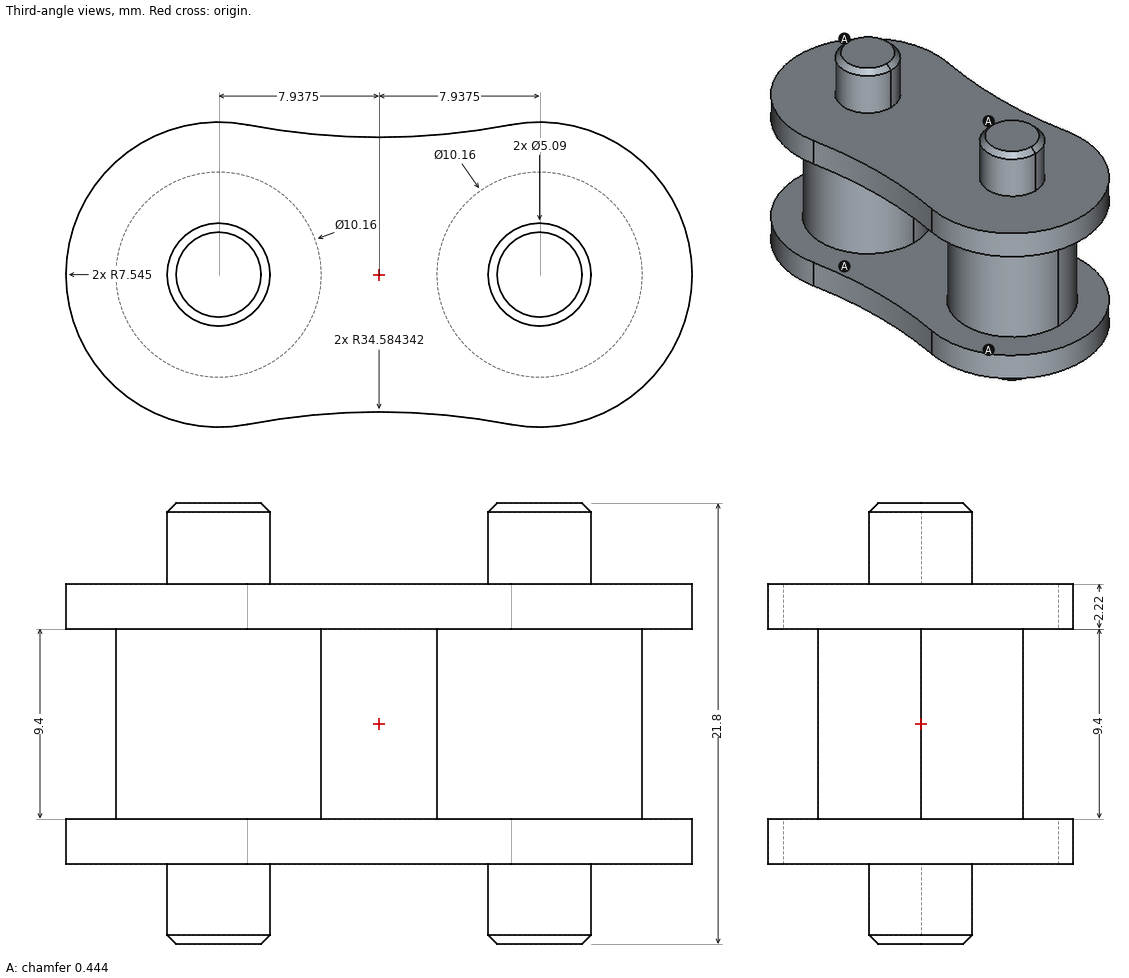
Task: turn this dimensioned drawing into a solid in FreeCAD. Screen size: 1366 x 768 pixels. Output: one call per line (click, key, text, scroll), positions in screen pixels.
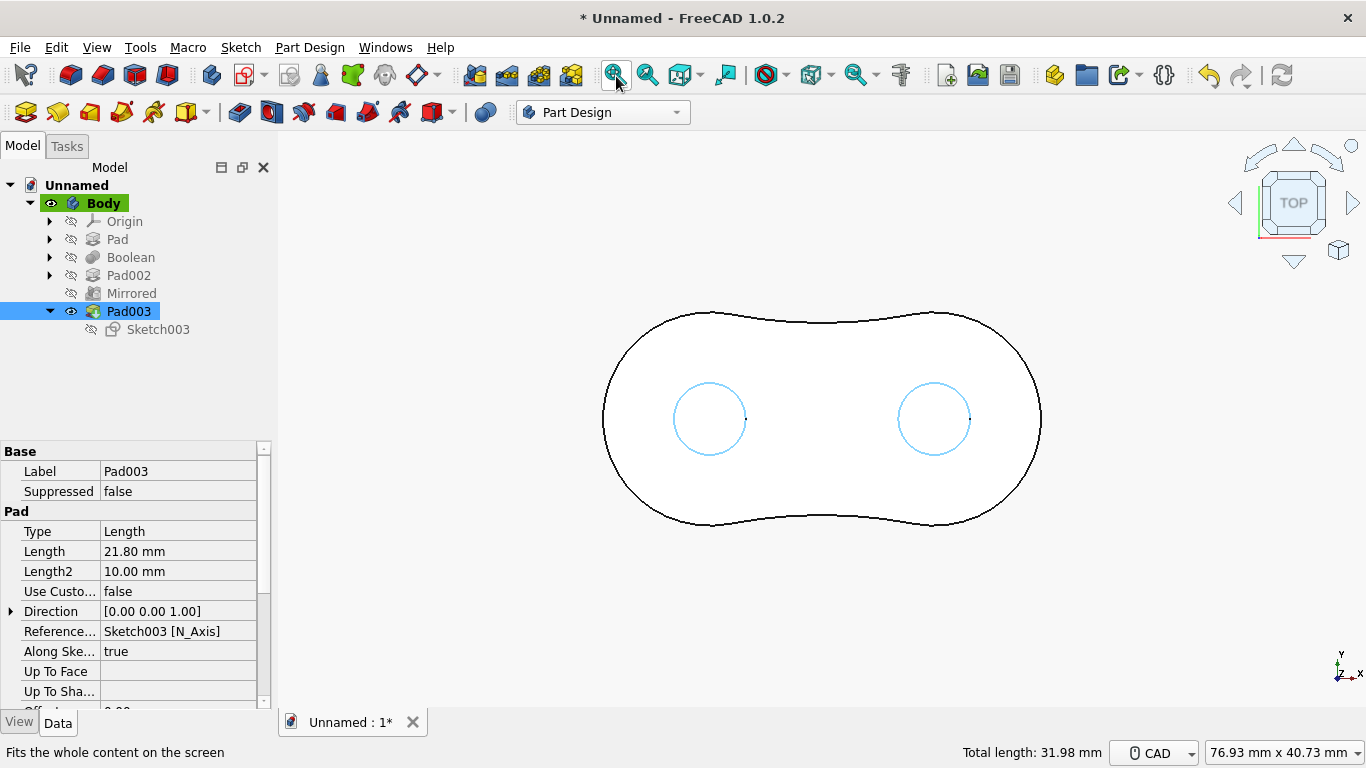
key(1)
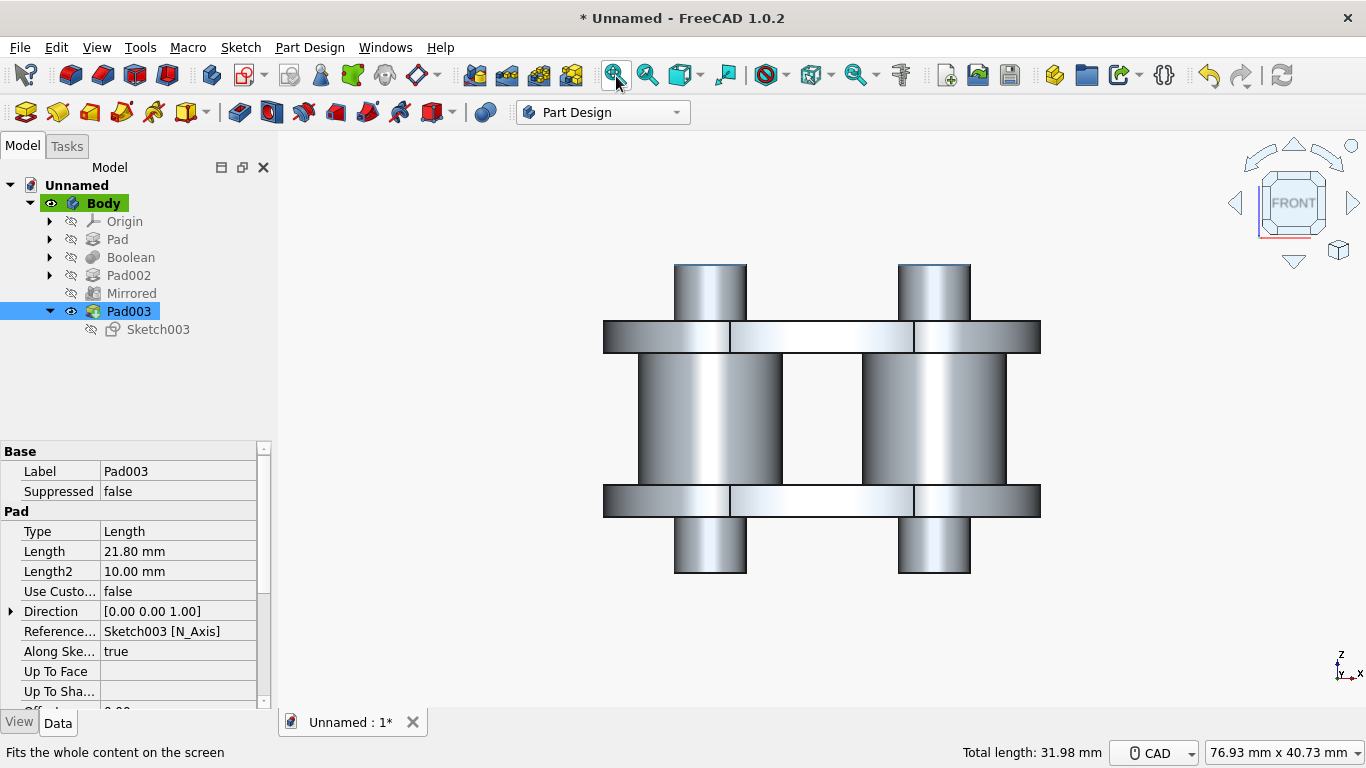
click(905, 572, ctrl)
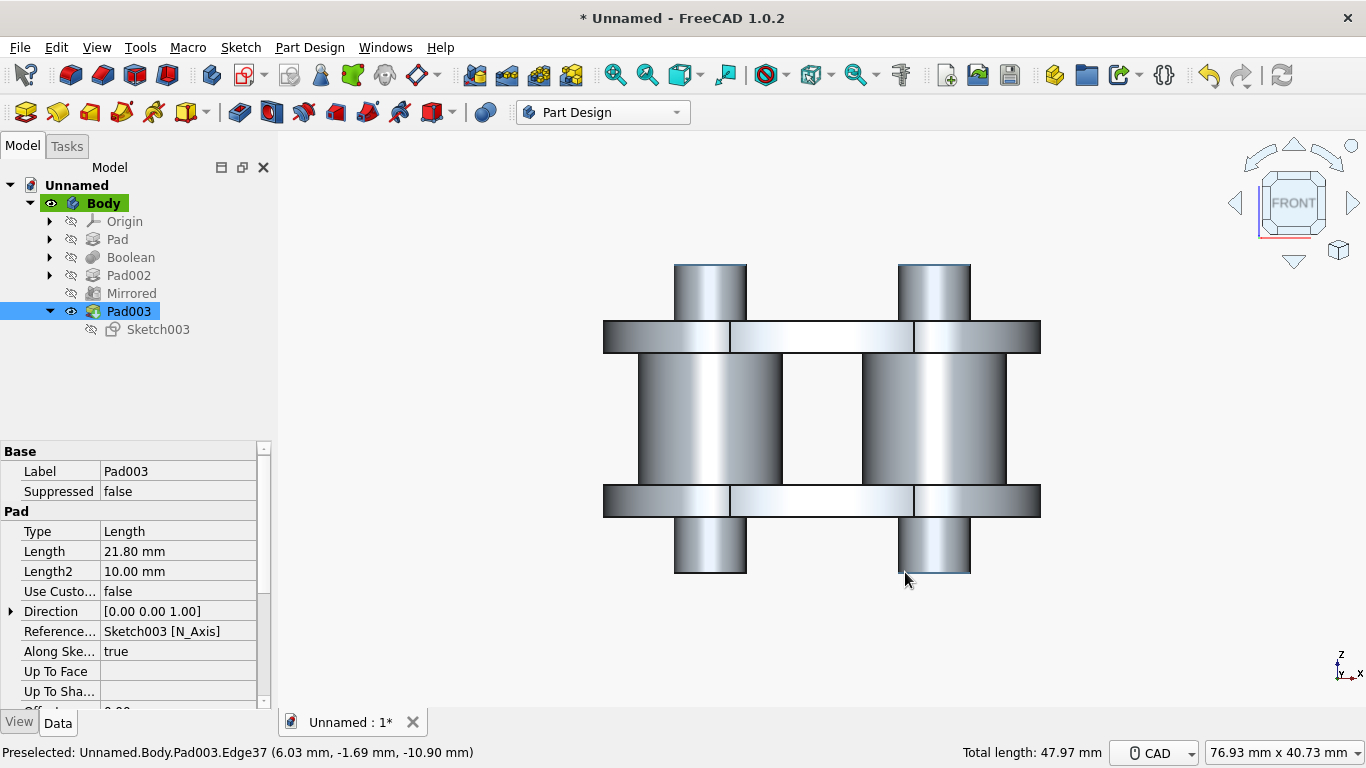
click(681, 572, ctrl)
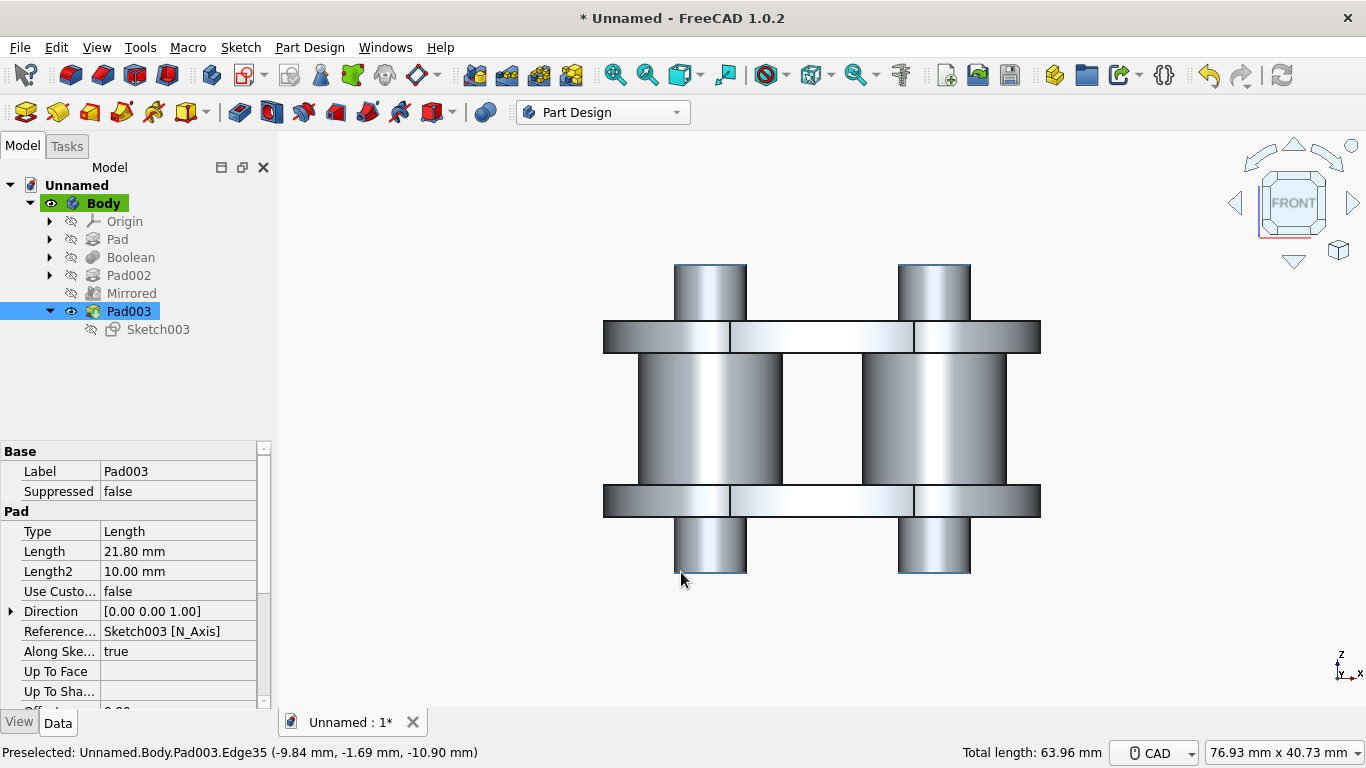
click(104, 76)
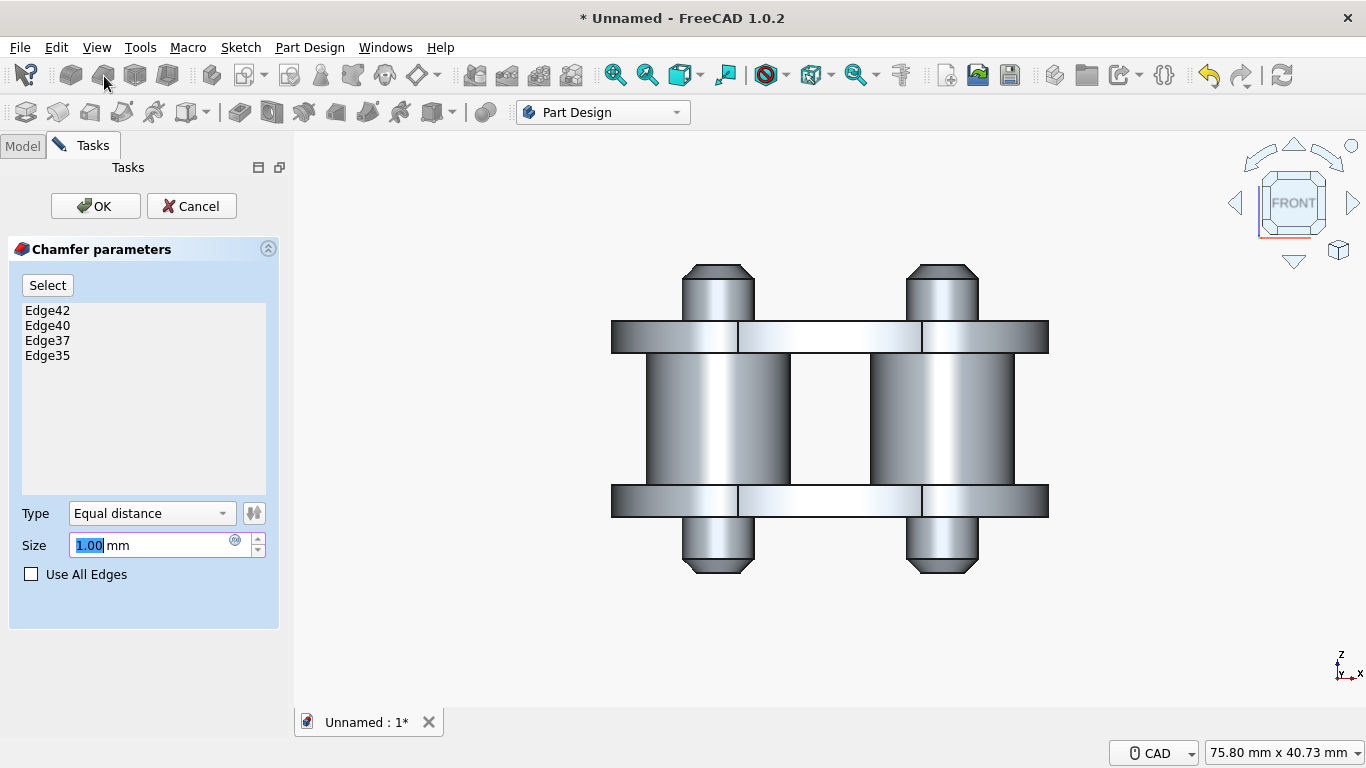
text(0.444)
key(Tab)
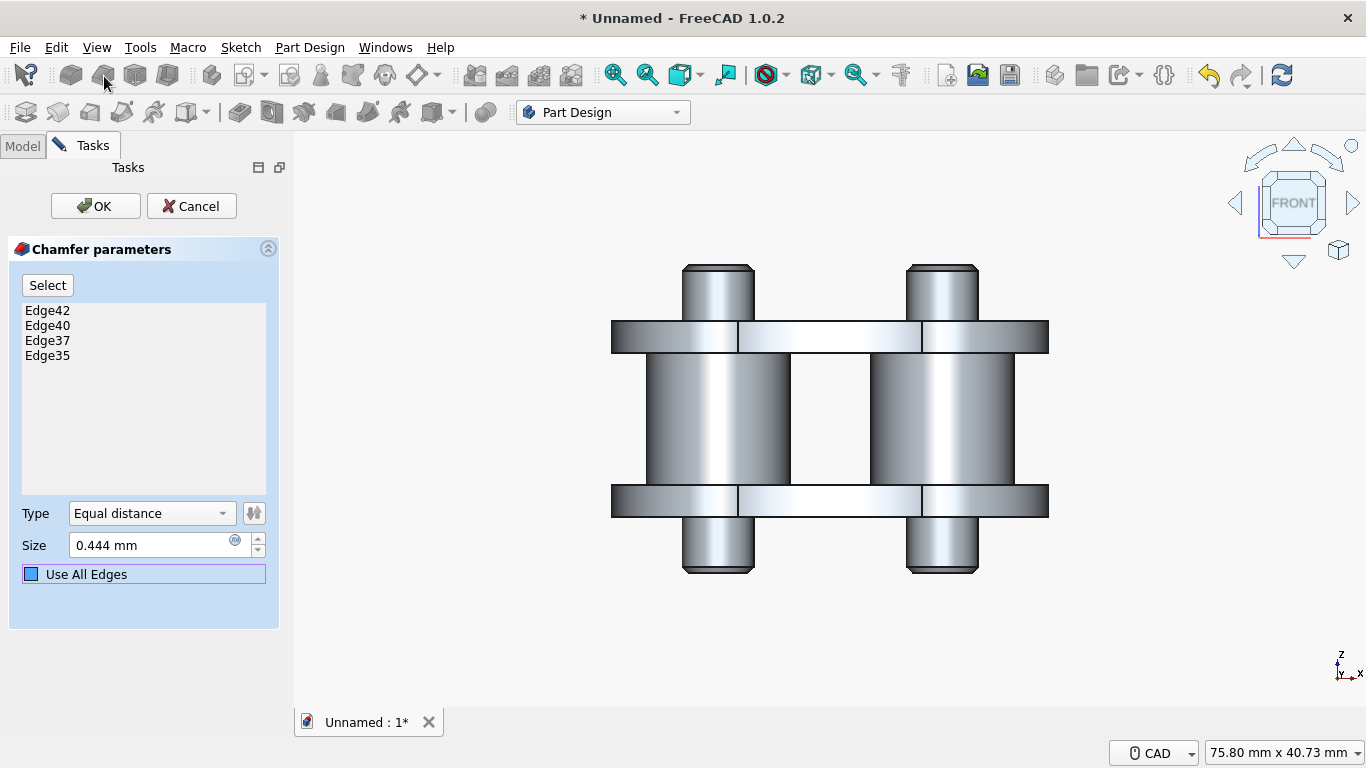
click(96, 206)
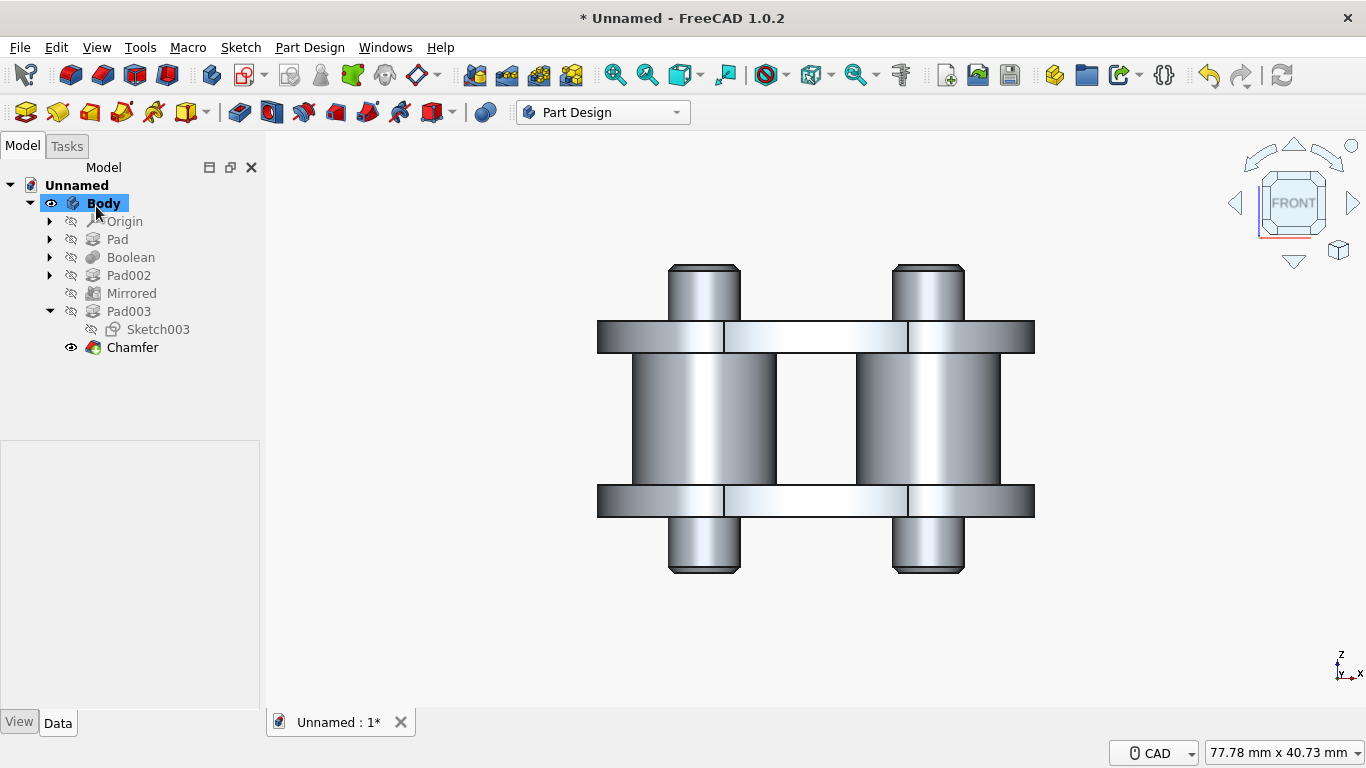
key(0)